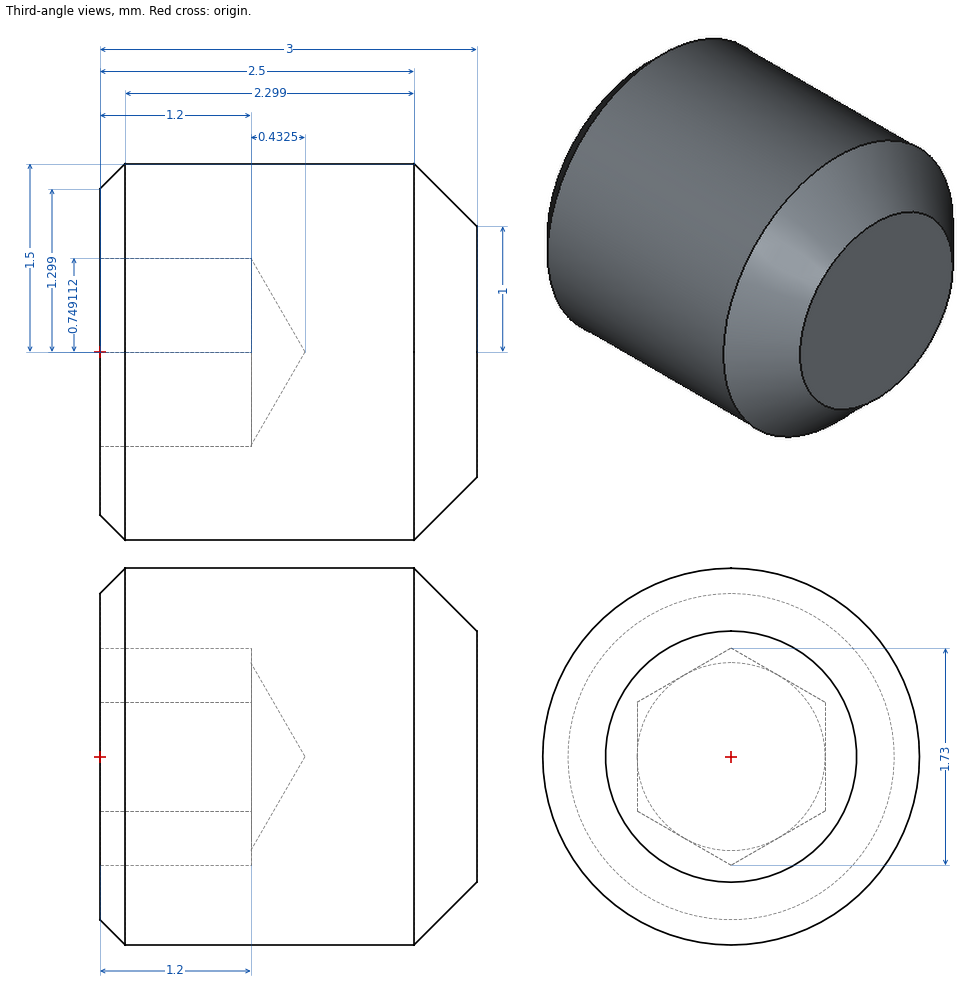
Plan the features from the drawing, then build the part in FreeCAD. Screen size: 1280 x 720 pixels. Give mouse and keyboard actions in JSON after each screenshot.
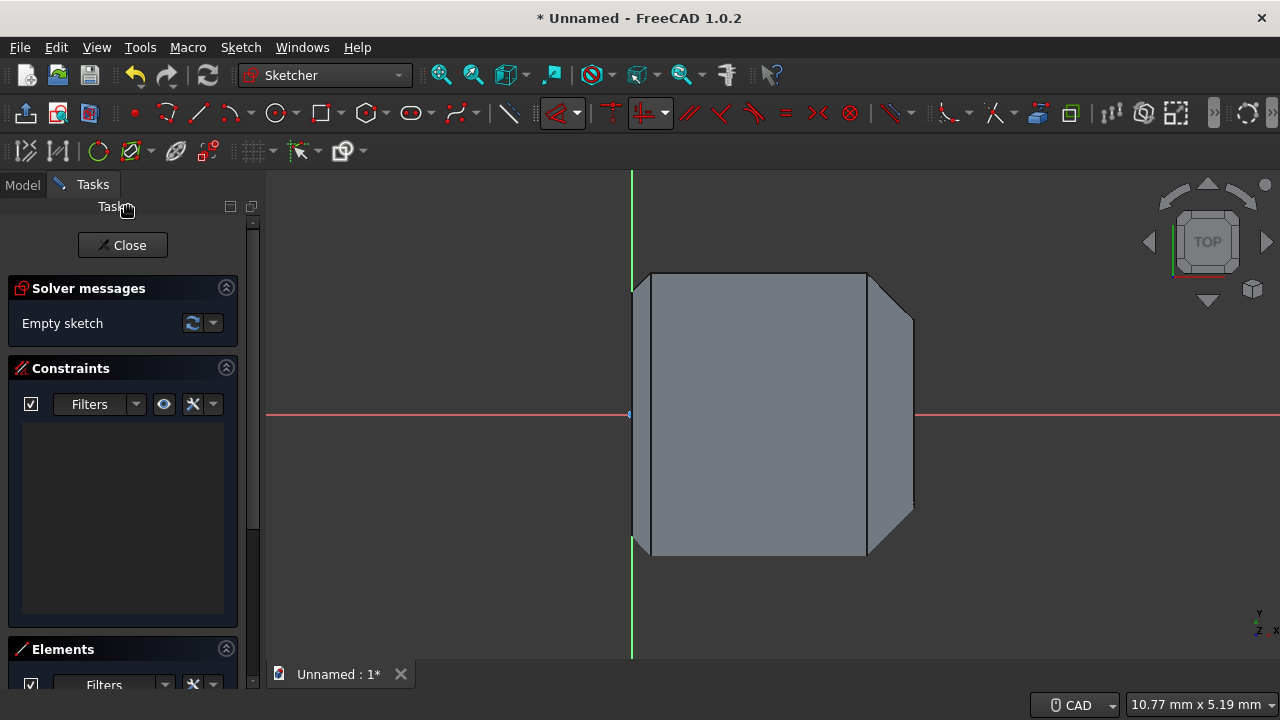
{"action": "left_click", "coordinate": [90, 114]}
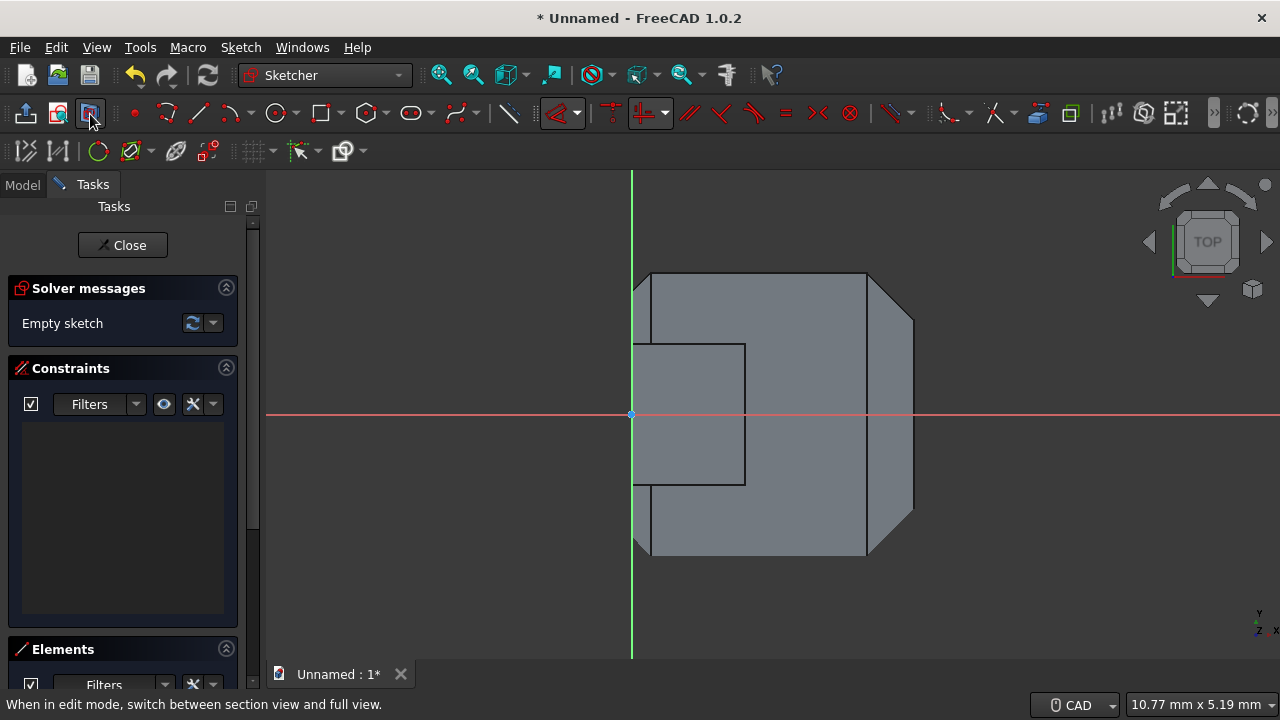
{"action": "scroll", "coordinate": [710, 368], "scroll_direction": "up", "scroll_amount": 7}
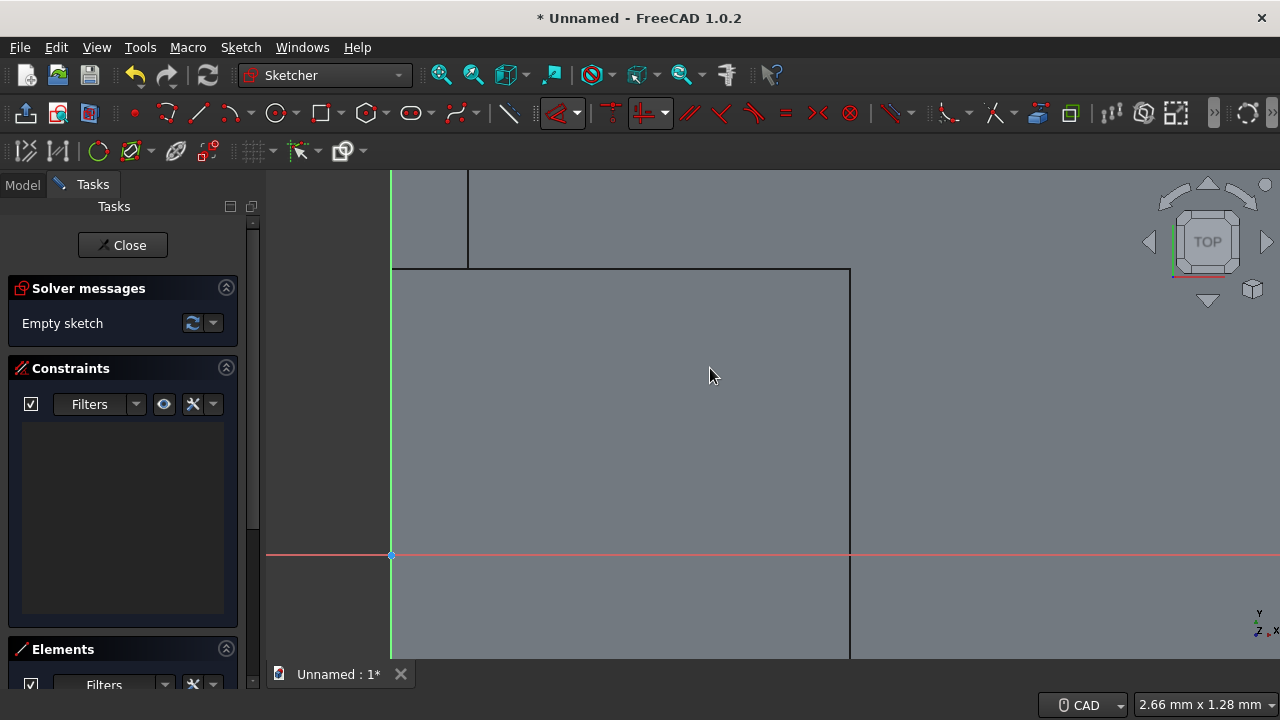
{"action": "left_click", "coordinate": [168, 114]}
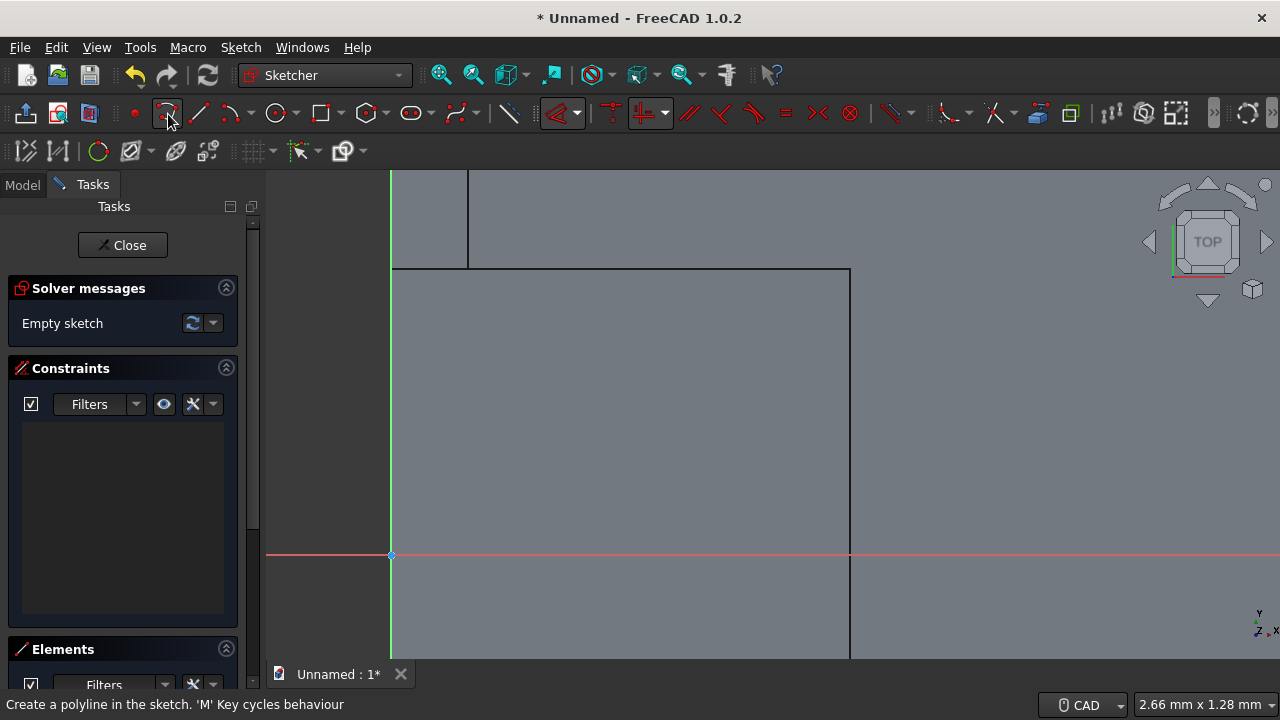
{"action": "left_click", "coordinate": [850, 555]}
{"action": "left_click", "coordinate": [1015, 546]}
{"action": "left_click", "coordinate": [850, 269]}
{"action": "left_click", "coordinate": [850, 555]}
{"action": "key", "text": "Escape"}
{"action": "key", "text": "Escape"}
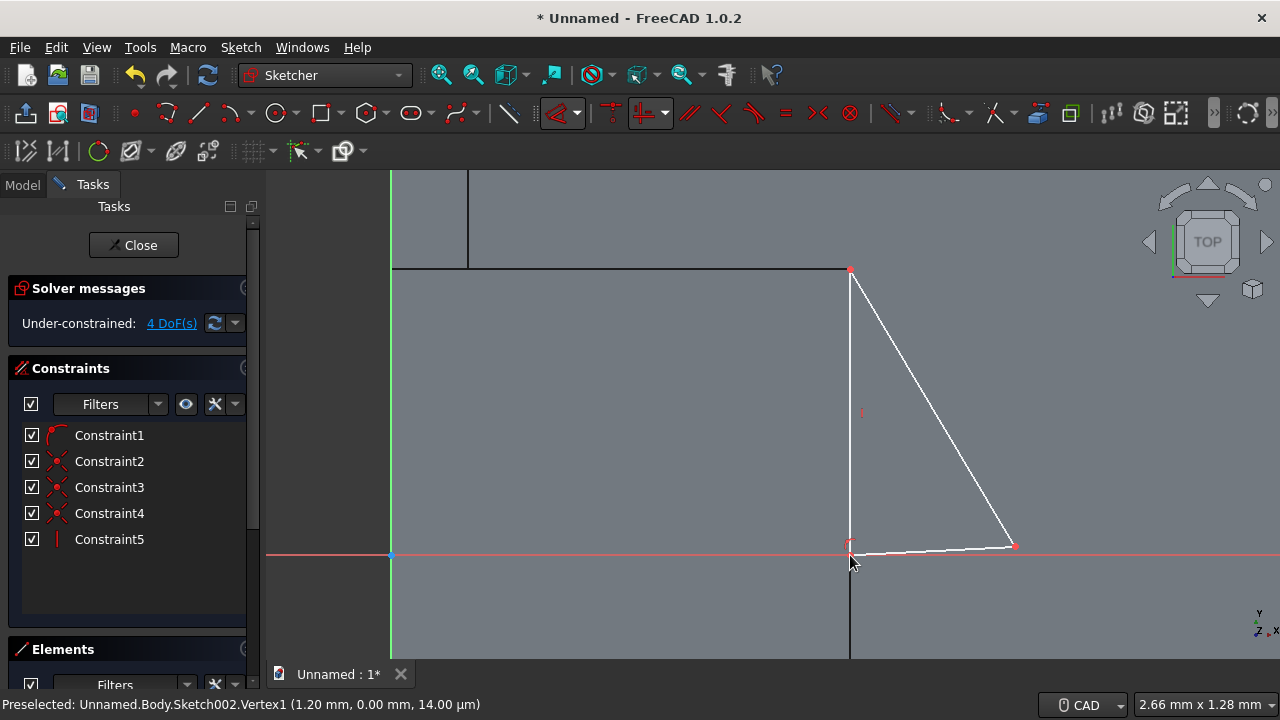
{"action": "left_click", "coordinate": [900, 553]}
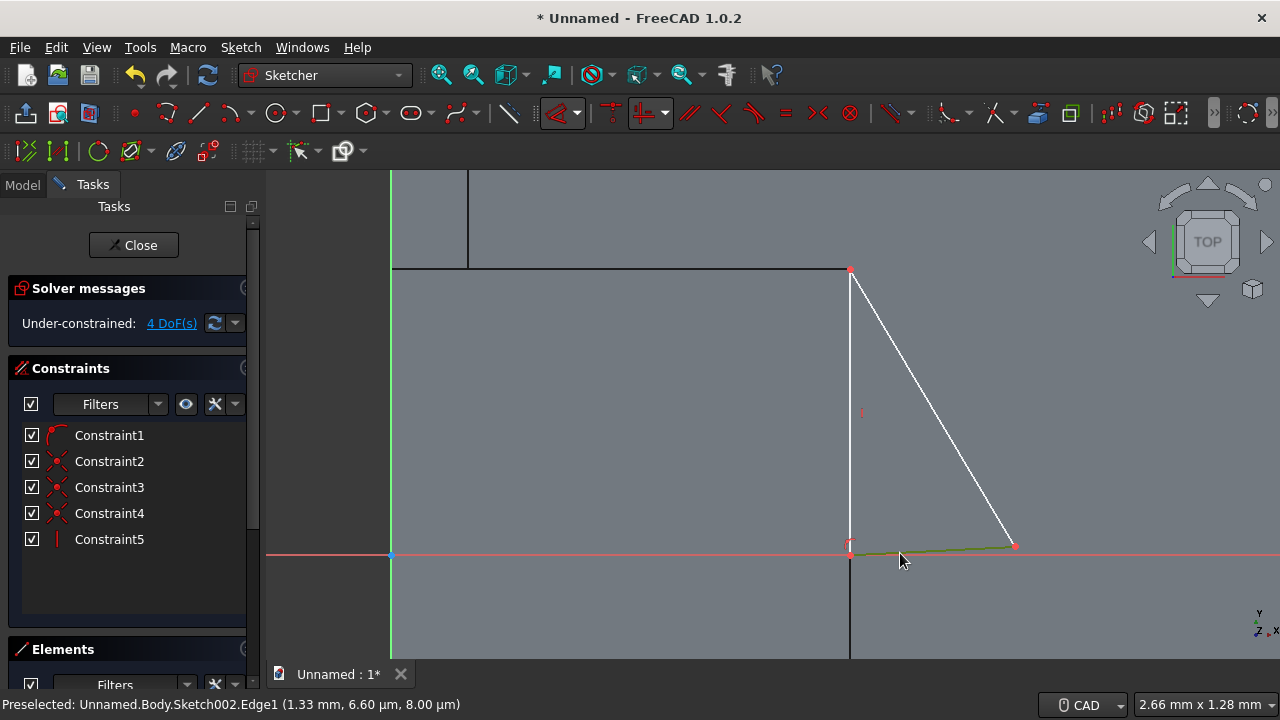
{"action": "left_click", "coordinate": [668, 114]}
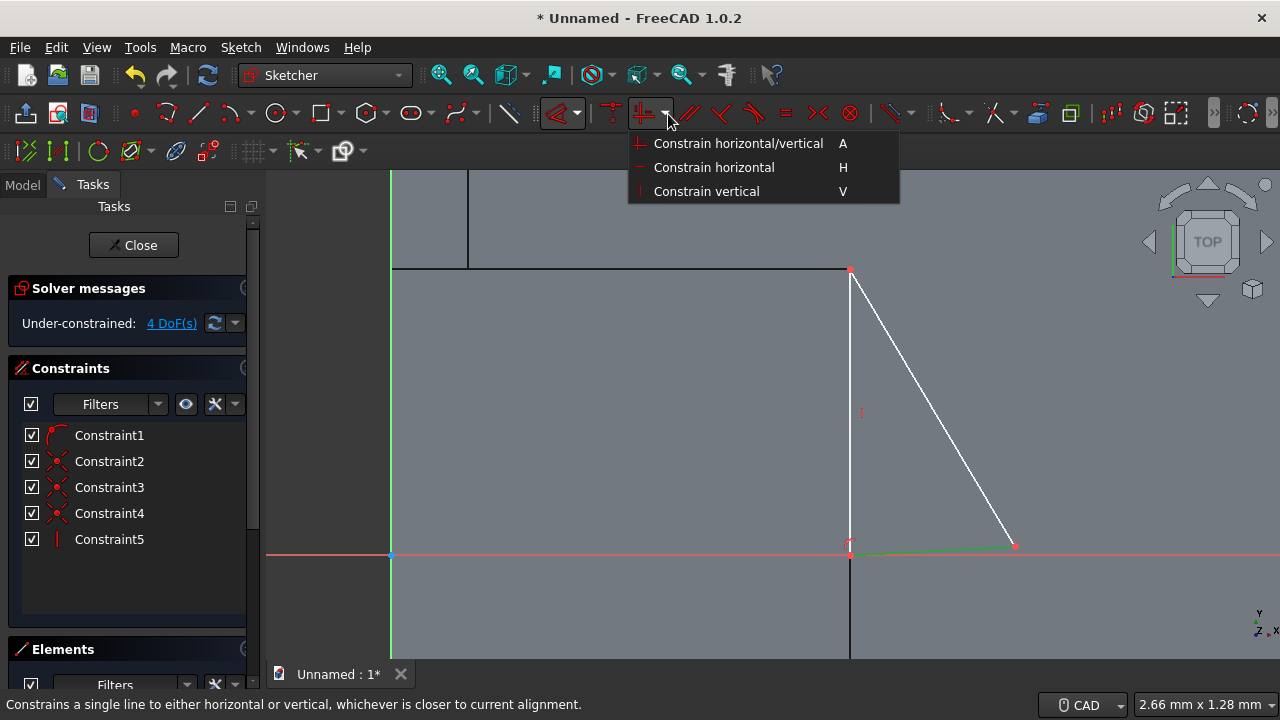
{"action": "left_click", "coordinate": [764, 167]}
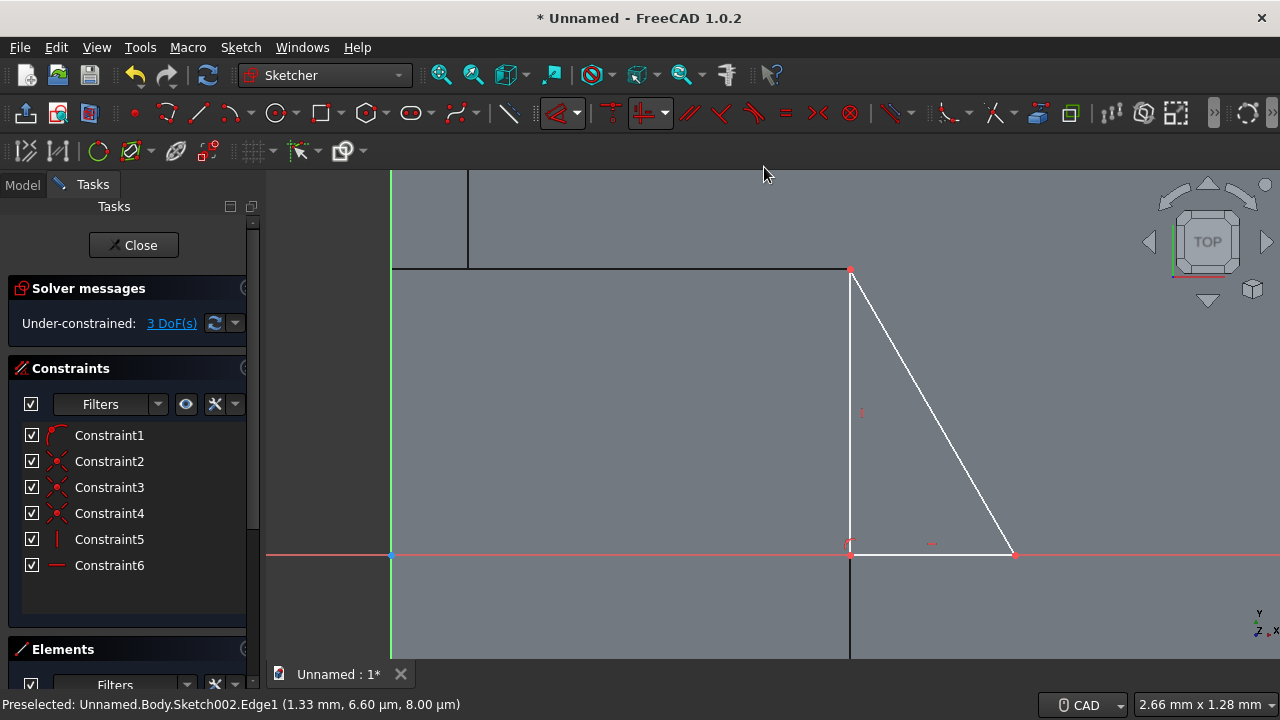
{"action": "left_click", "coordinate": [850, 555]}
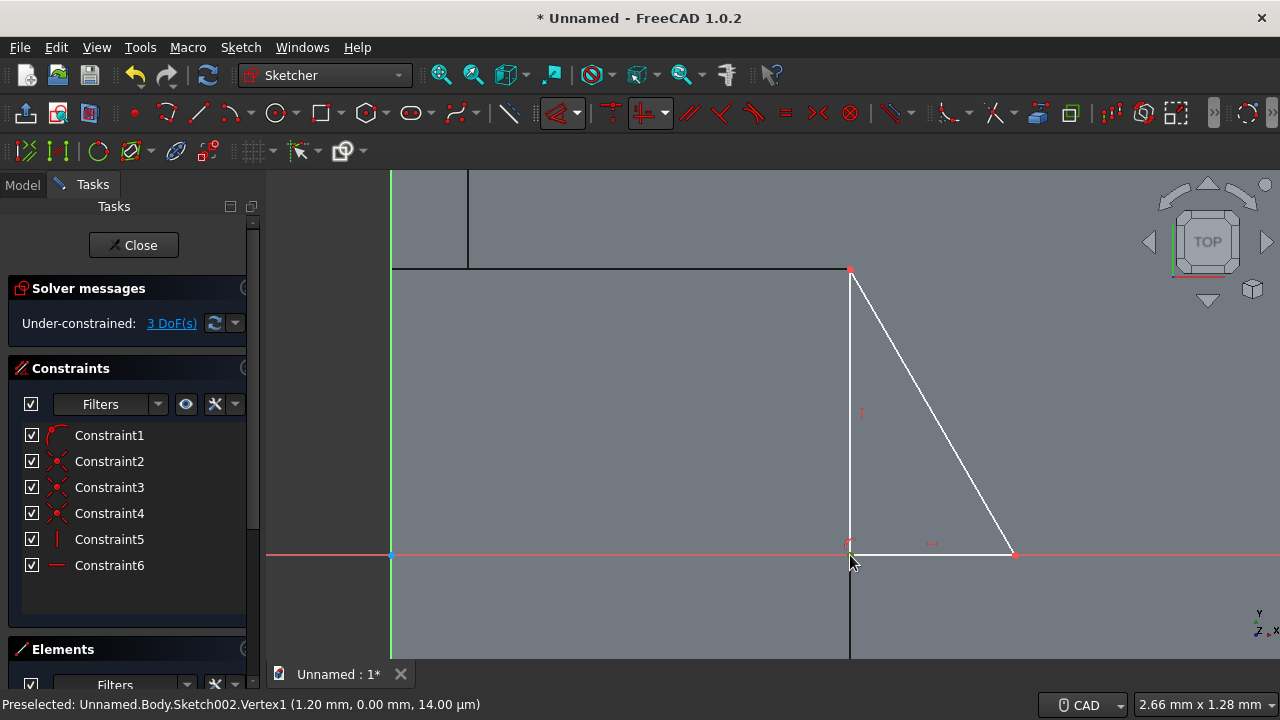
{"action": "key", "text": "l"}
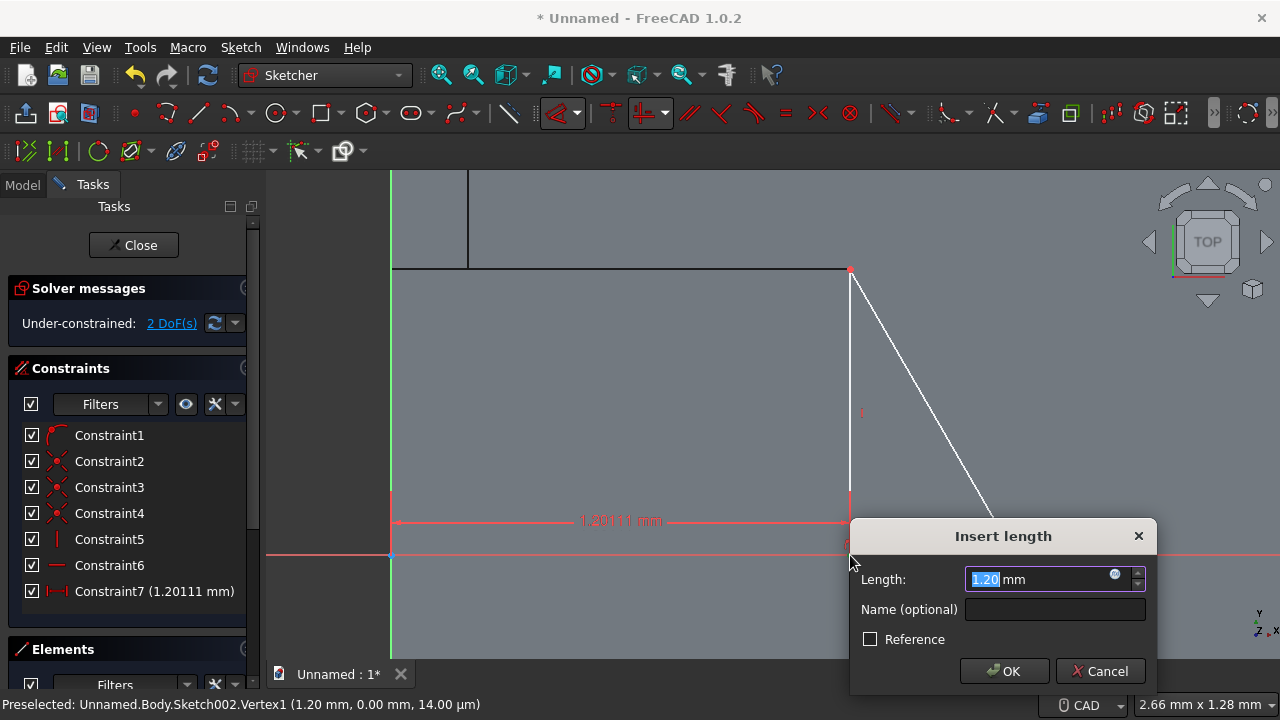
{"action": "type", "text": "1.2"}
{"action": "key", "text": "Return"}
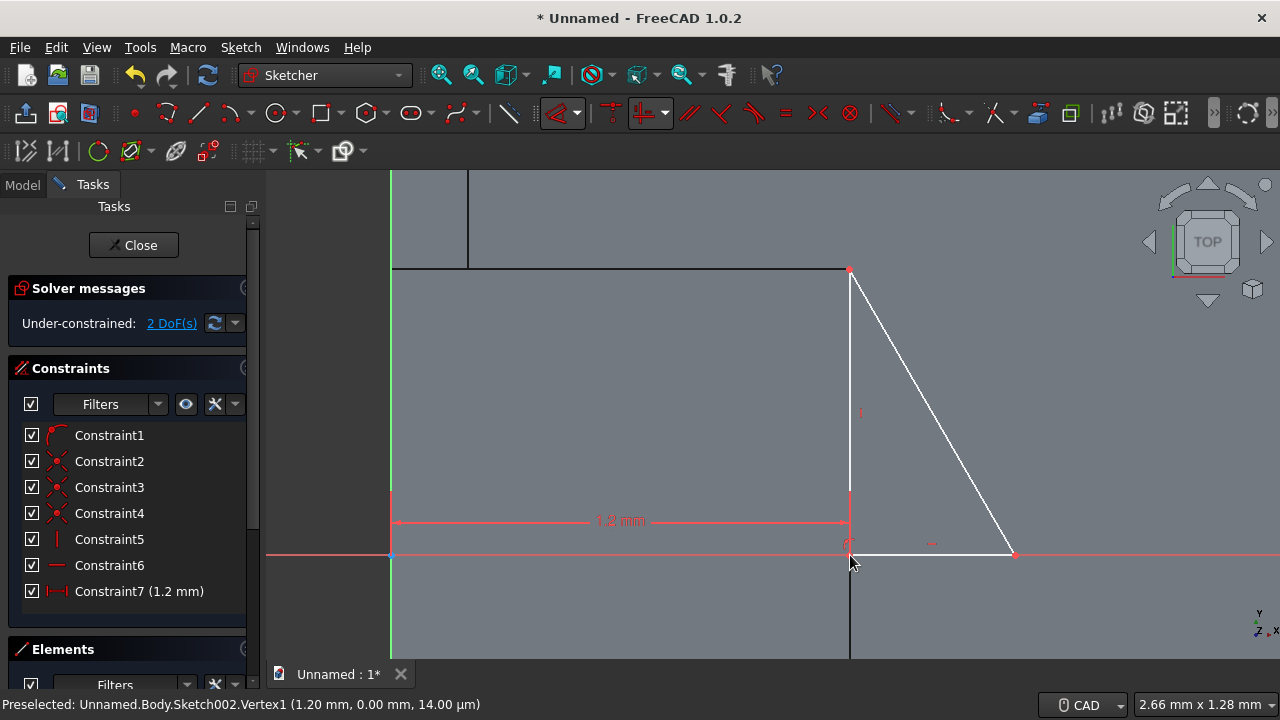
{"action": "left_click", "coordinate": [899, 555]}